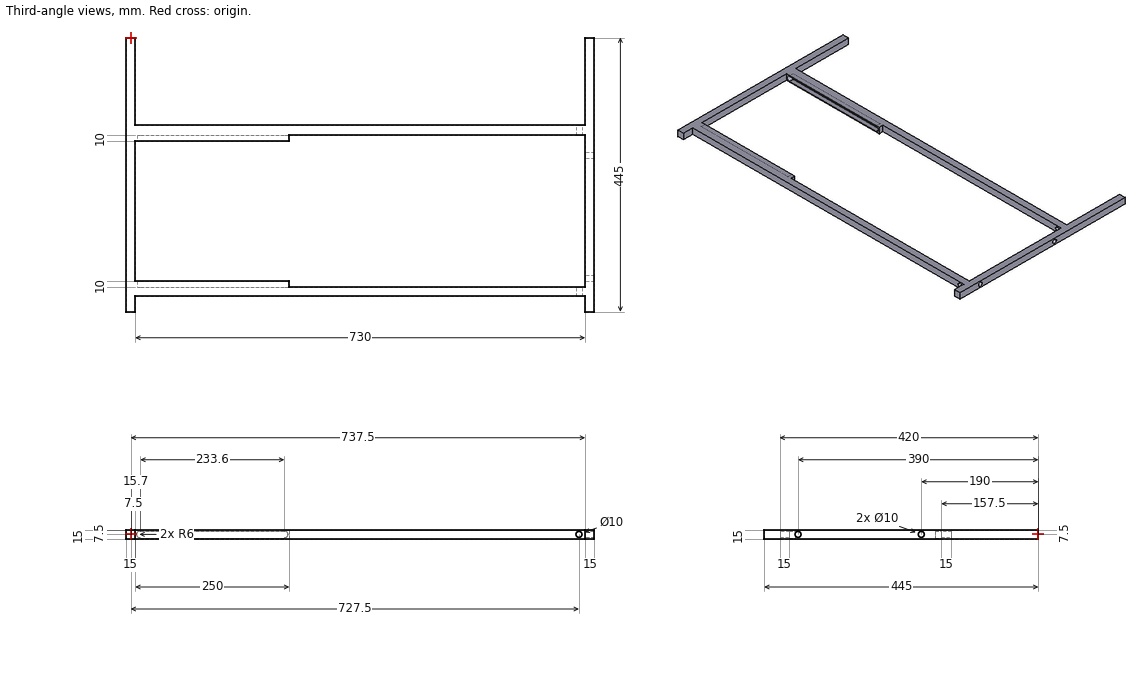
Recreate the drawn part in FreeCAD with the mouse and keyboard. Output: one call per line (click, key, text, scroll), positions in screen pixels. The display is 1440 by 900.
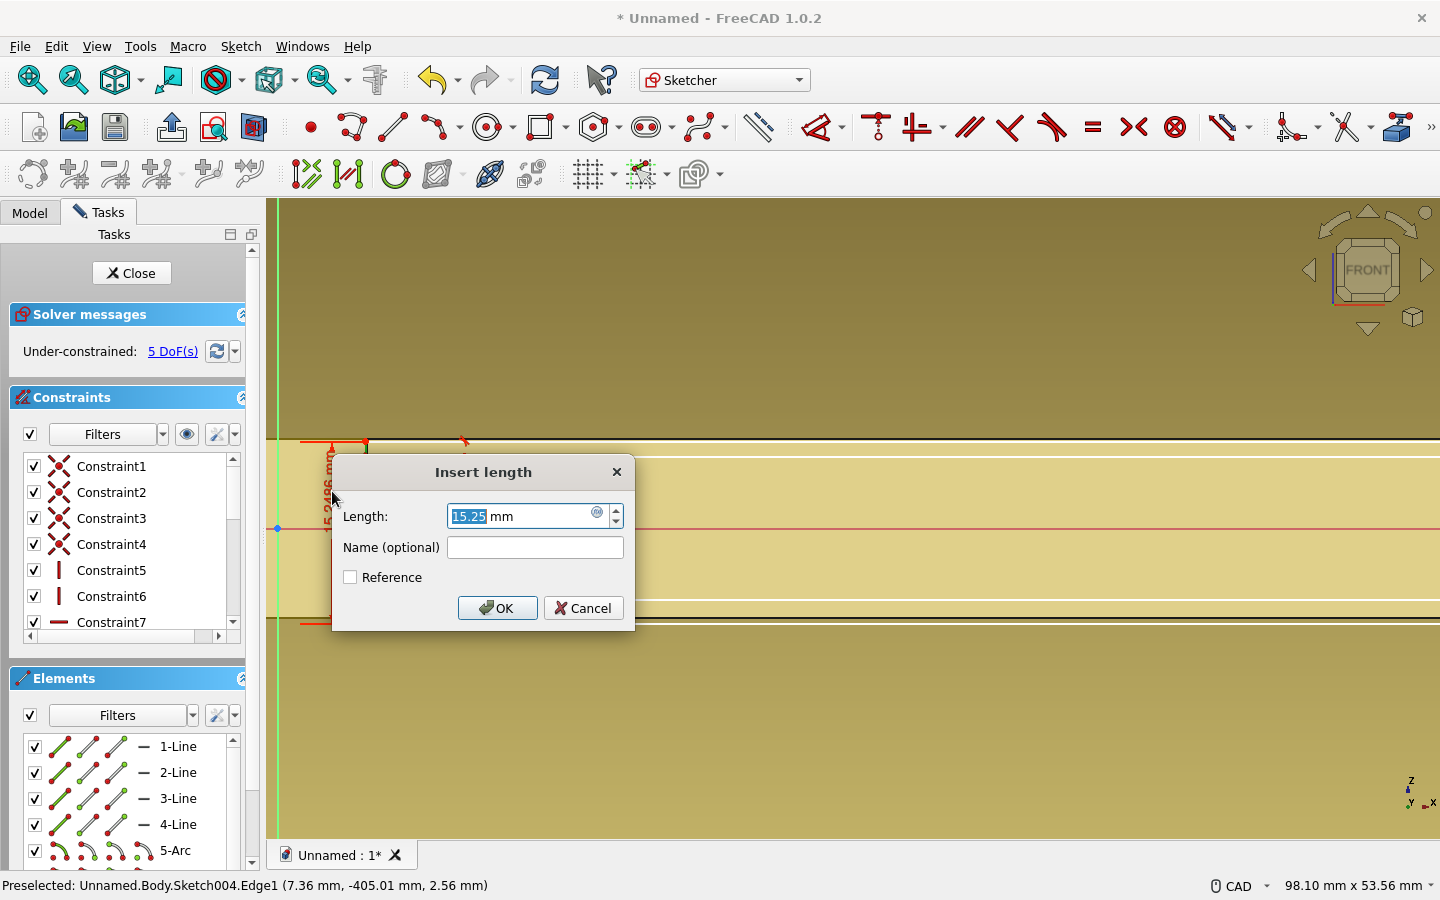
text(15)
key(Return)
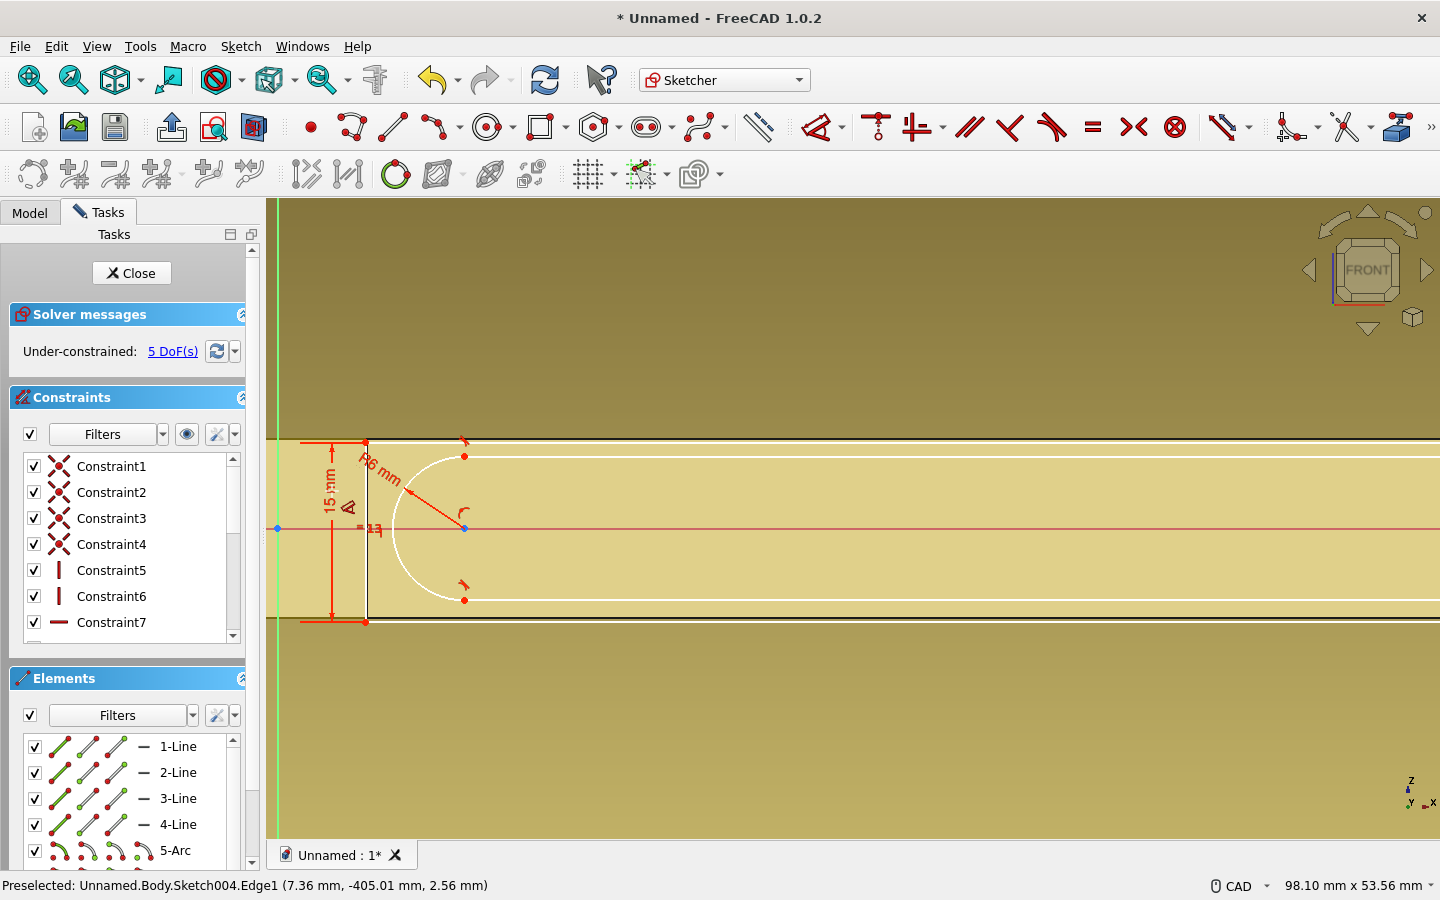
click(1264, 622)
click(820, 656)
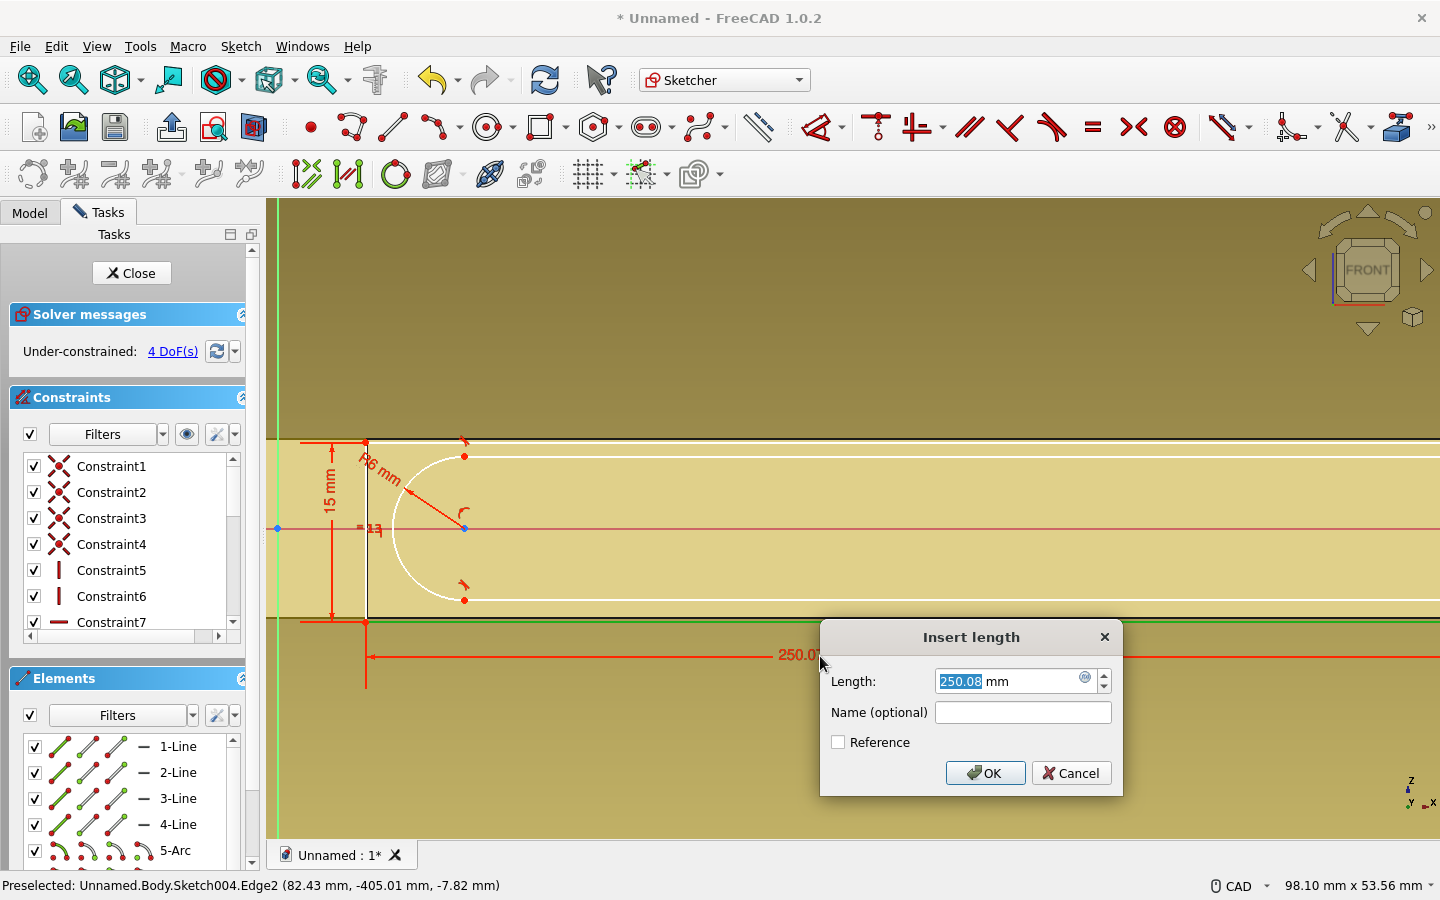
text(250)
key(Return)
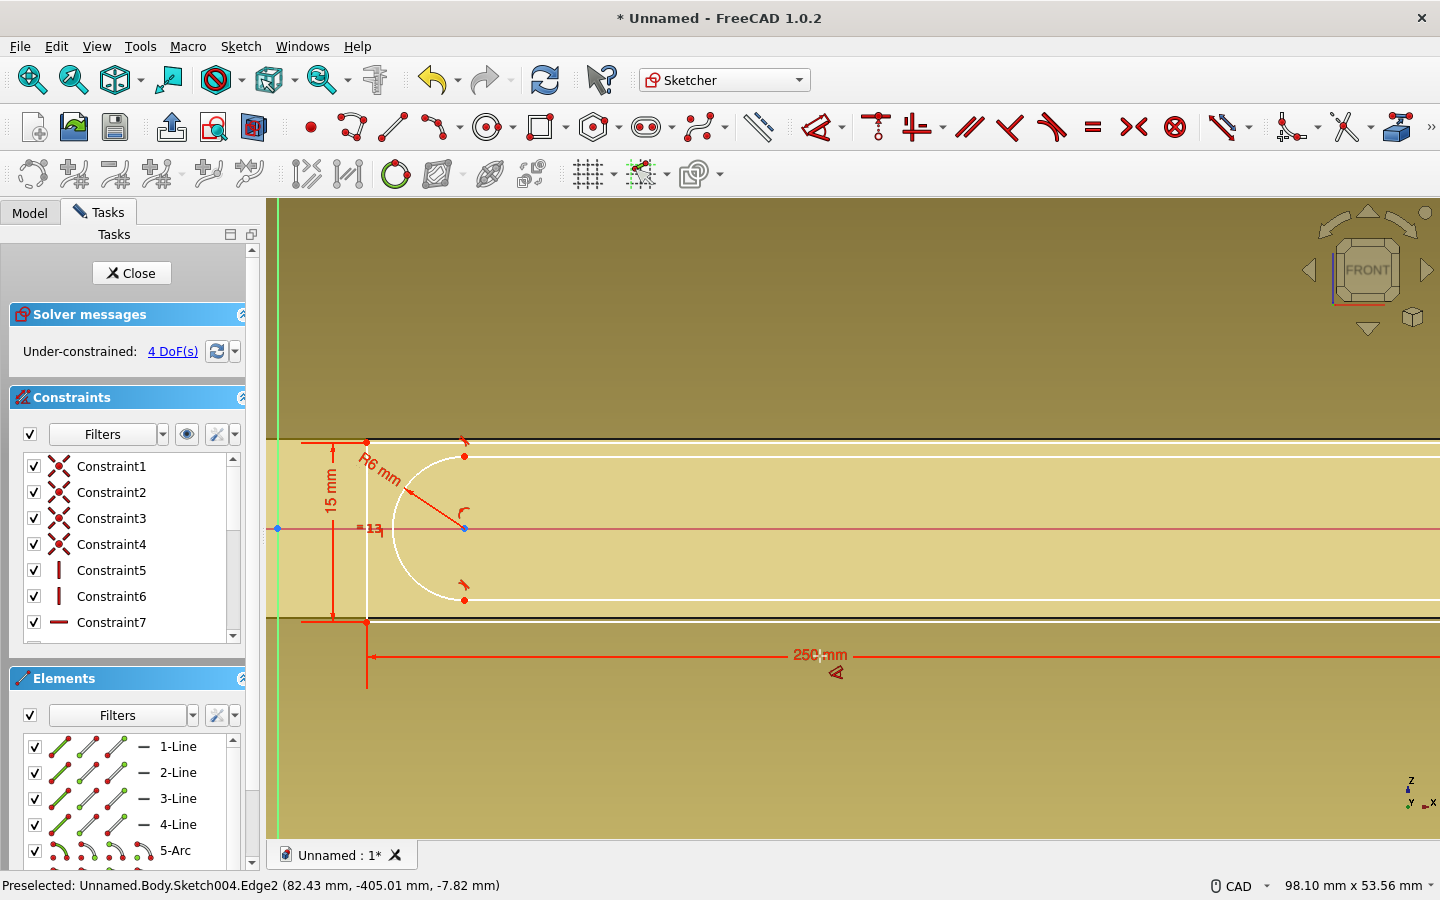
click(367, 443)
click(330, 409)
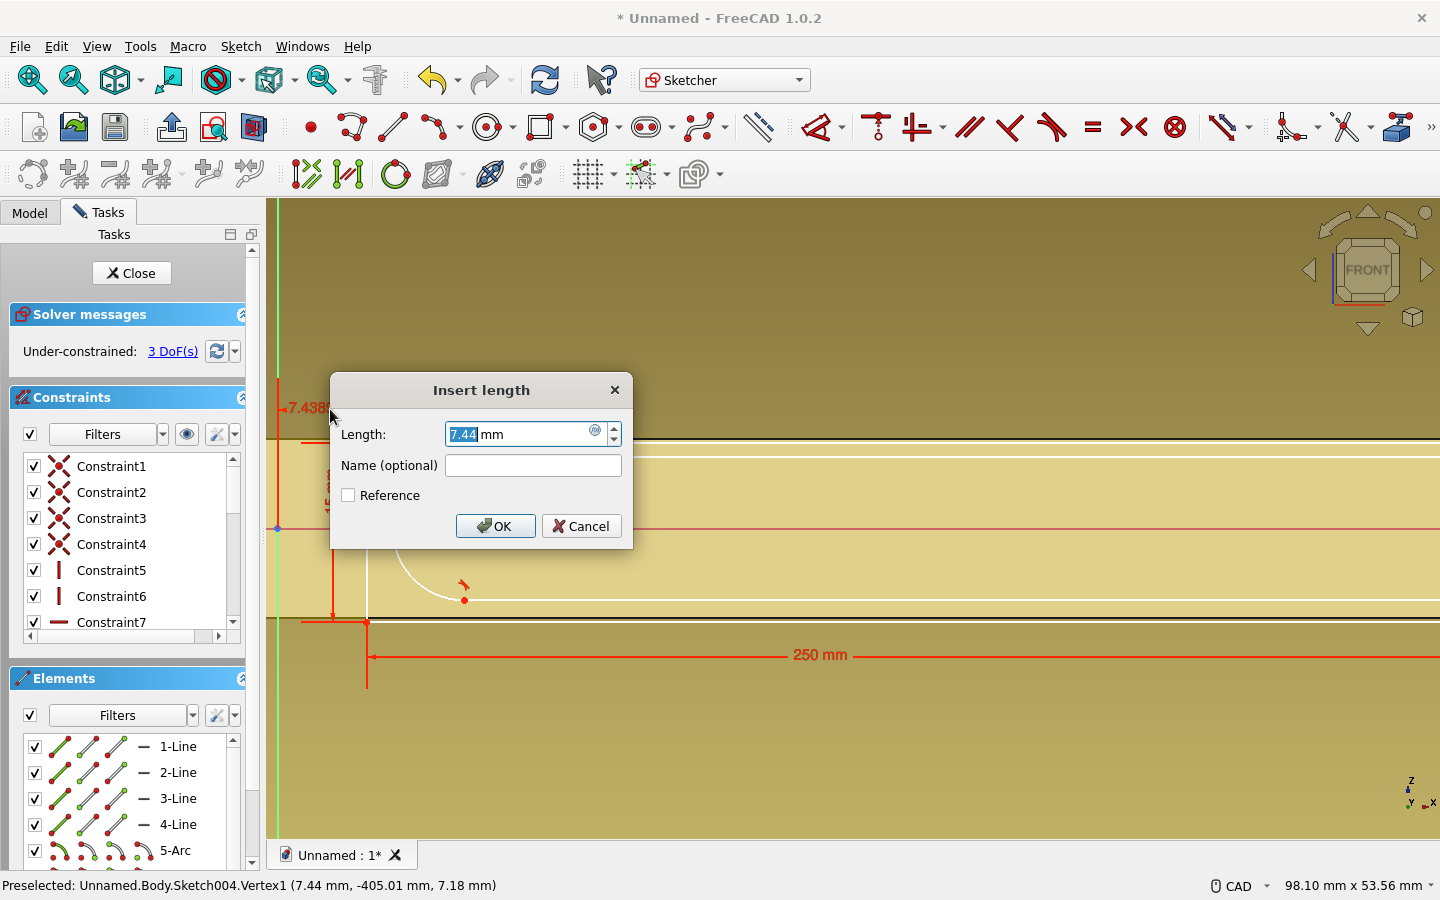
text(7.5)
key(Return)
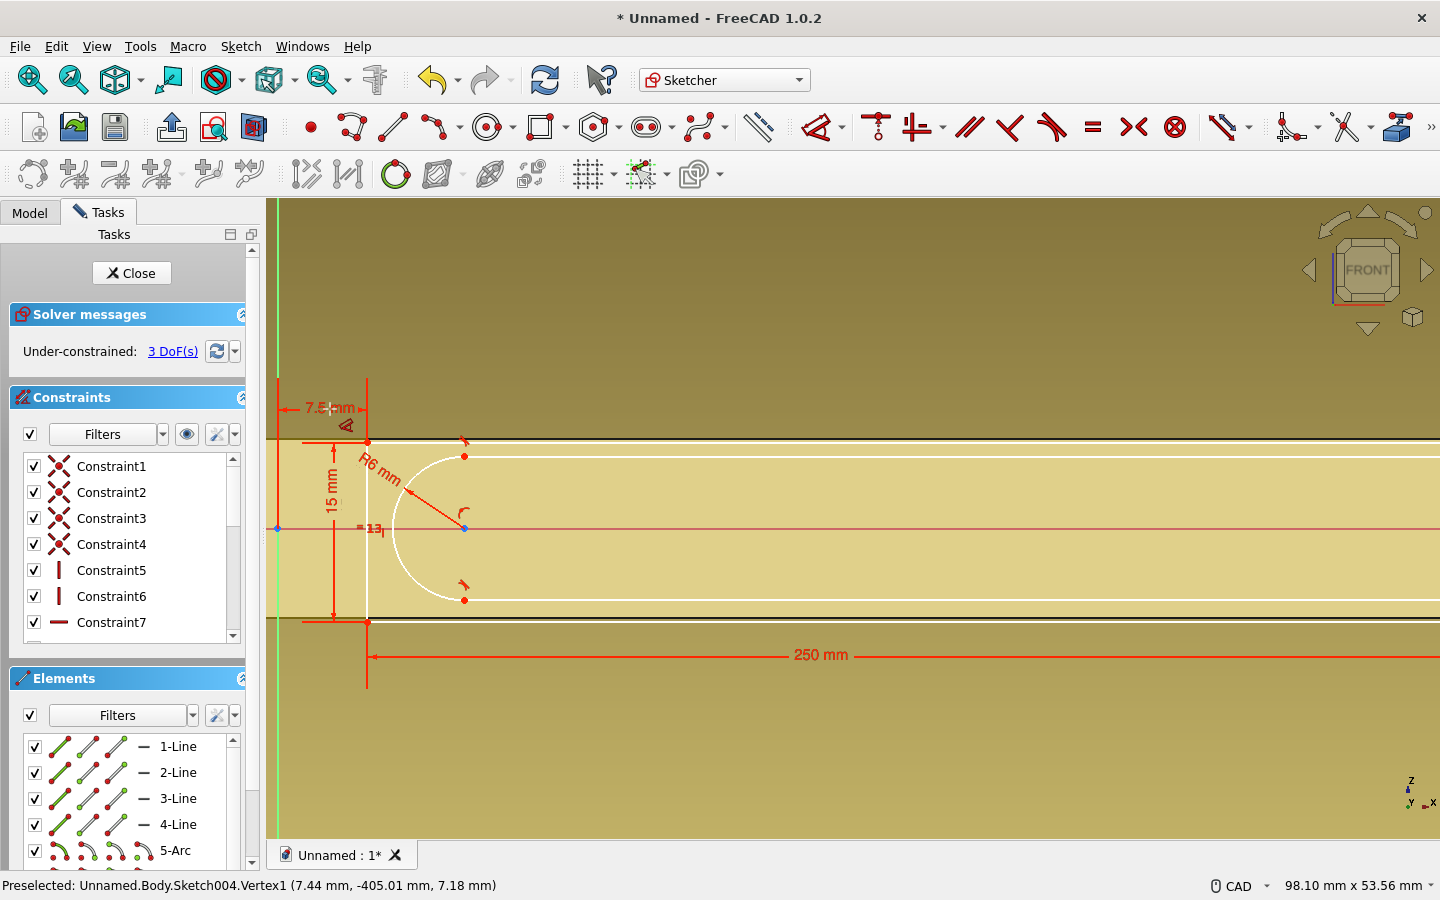
click(367, 443)
click(401, 466)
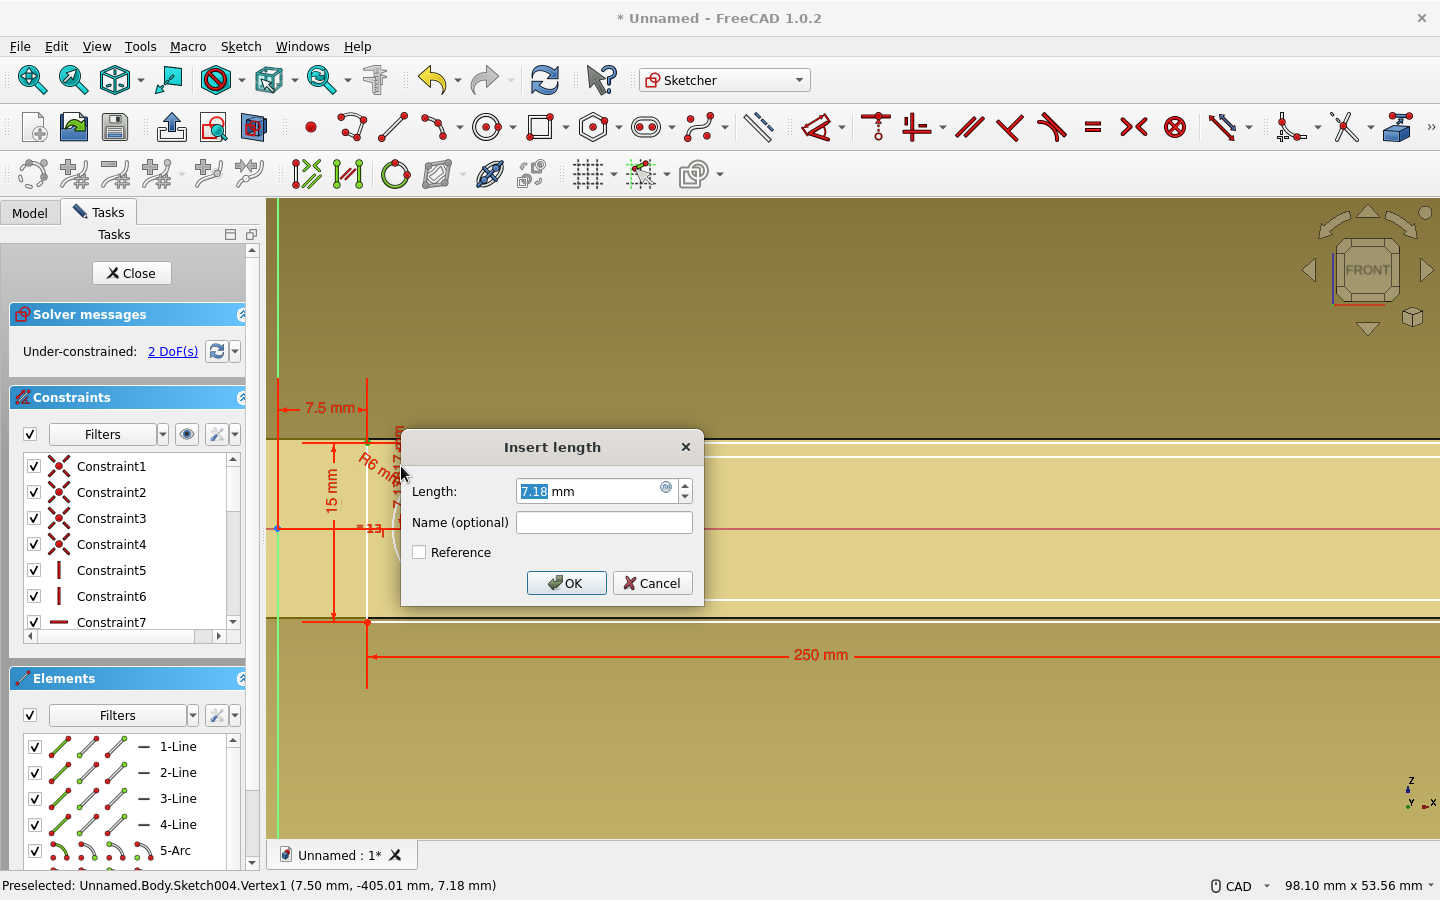
text(7.5)
key(Return)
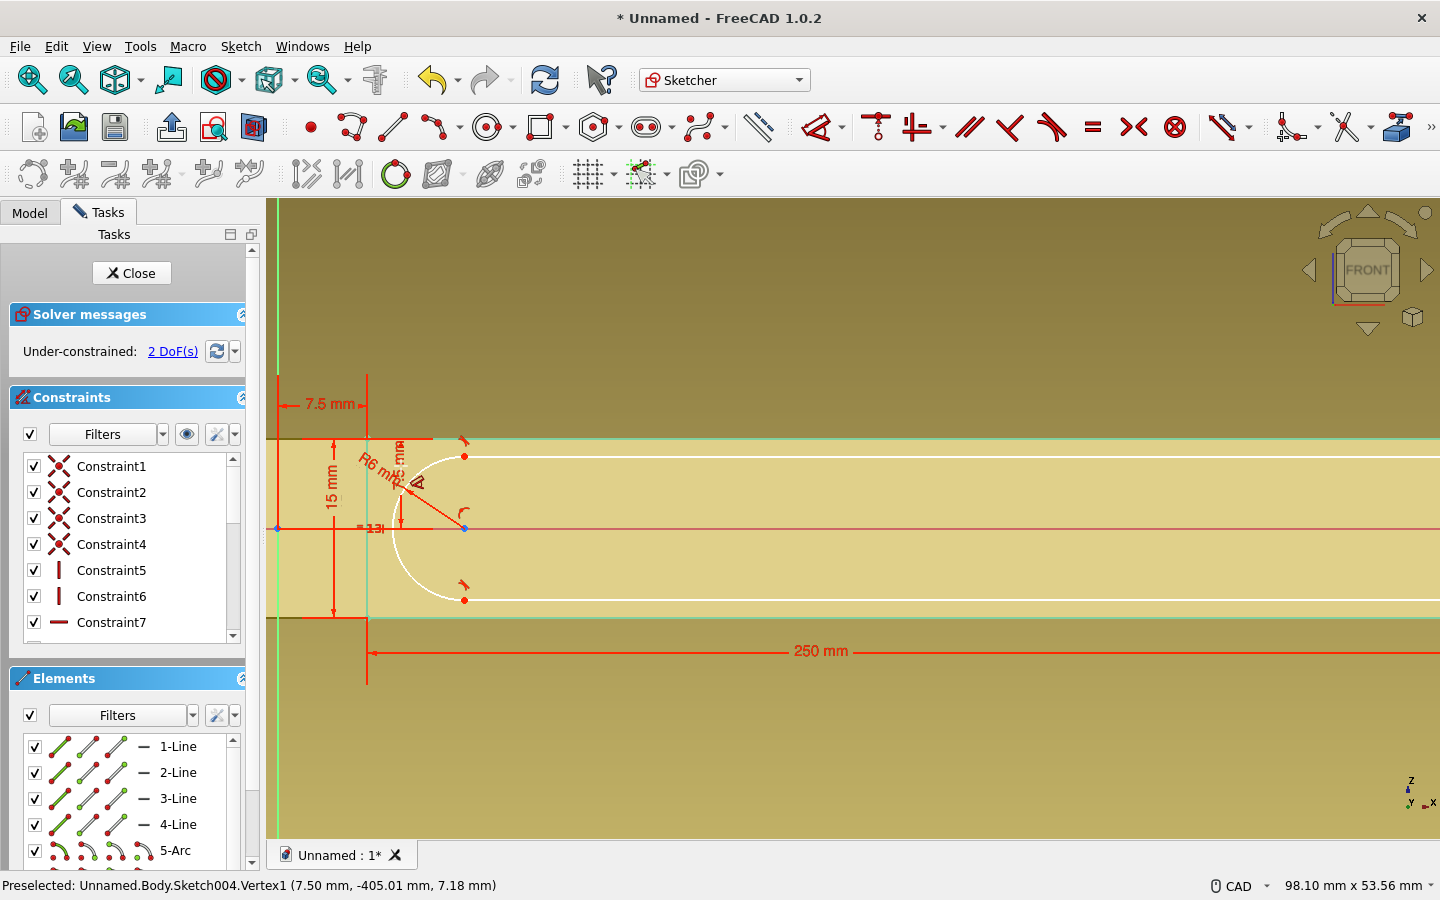
click(1023, 457)
click(870, 423)